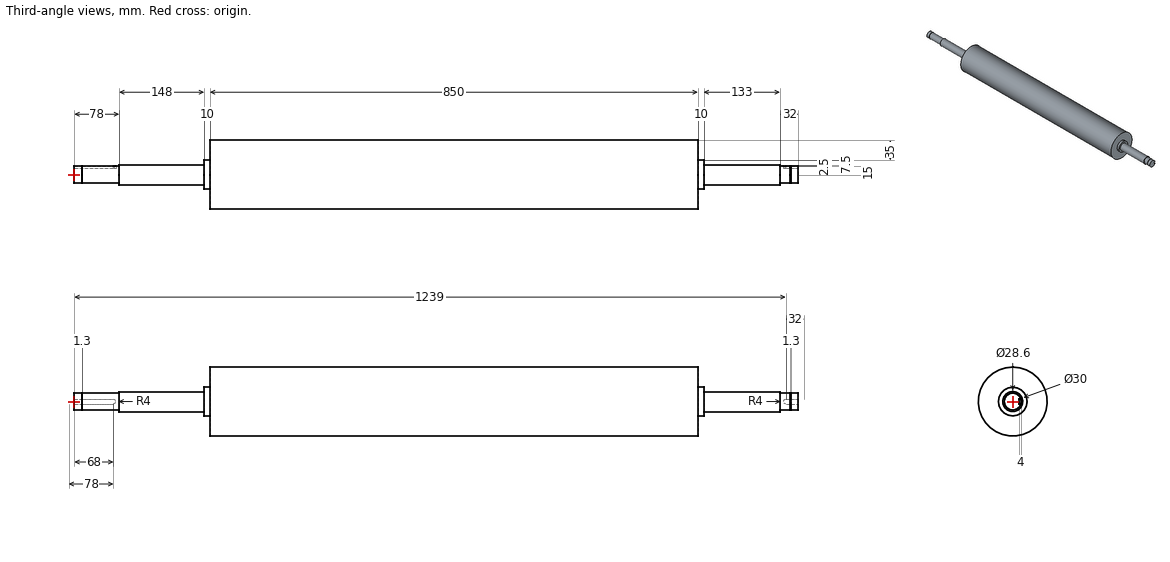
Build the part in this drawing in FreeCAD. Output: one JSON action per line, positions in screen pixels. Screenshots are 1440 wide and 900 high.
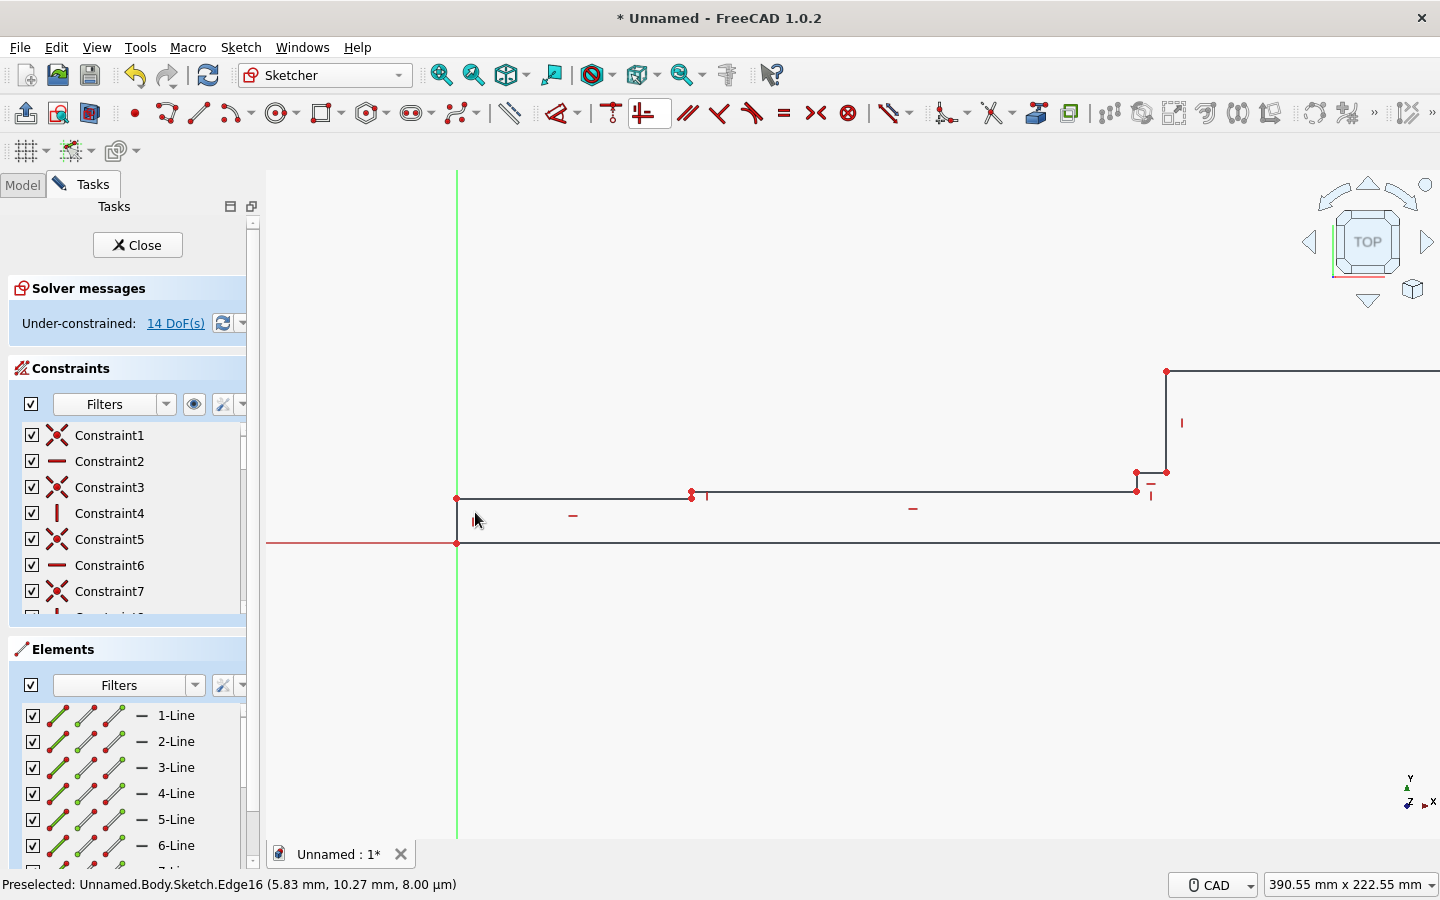
{"action": "scroll", "coordinate": [474, 515], "scroll_direction": "down", "scroll_amount": 9}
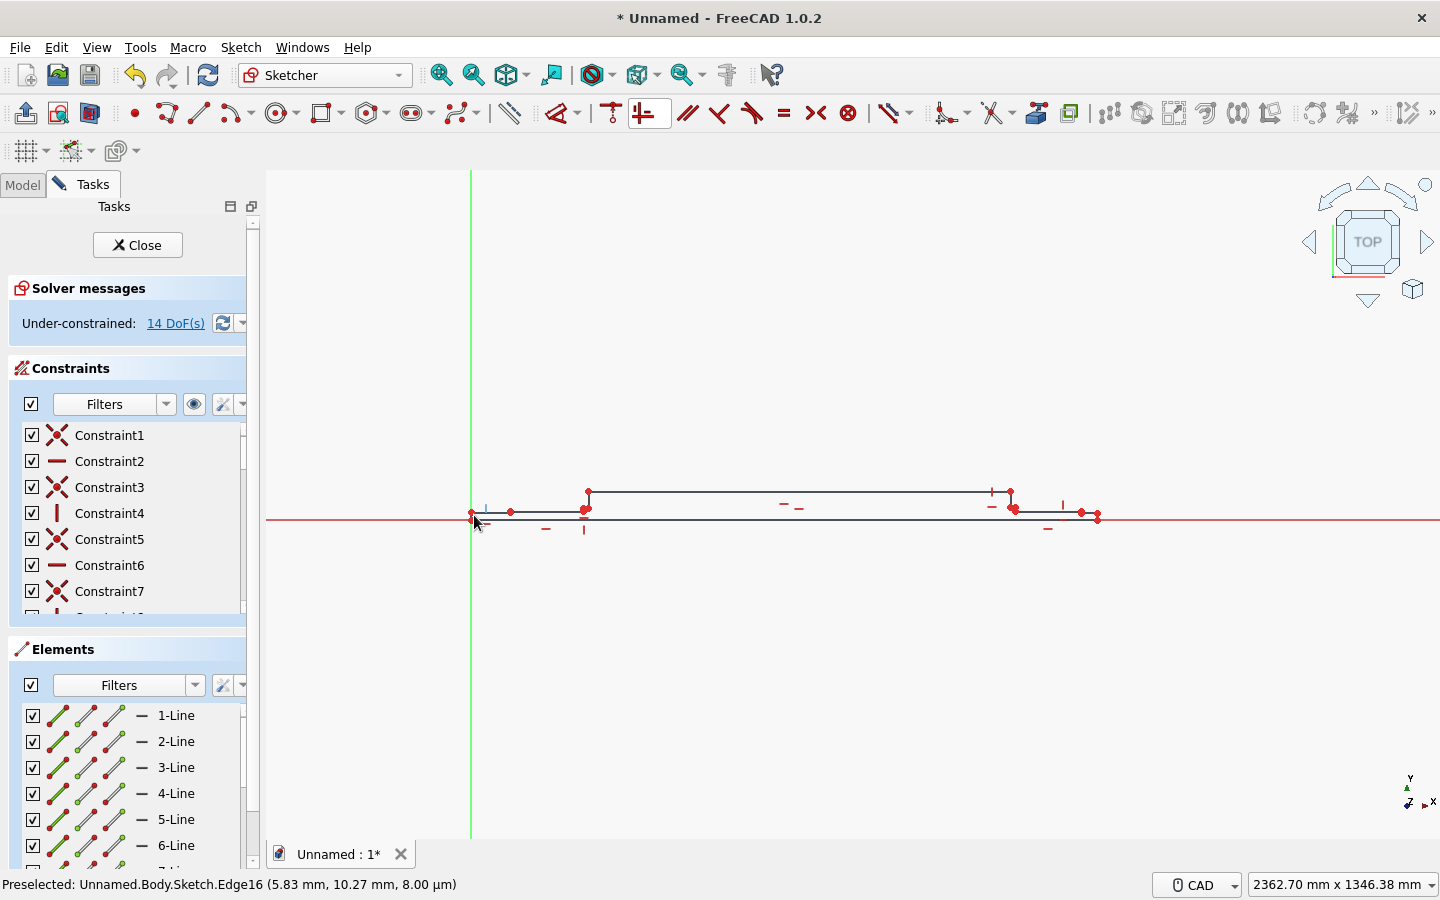
{"action": "scroll", "coordinate": [1098, 518], "scroll_direction": "up", "scroll_amount": 10}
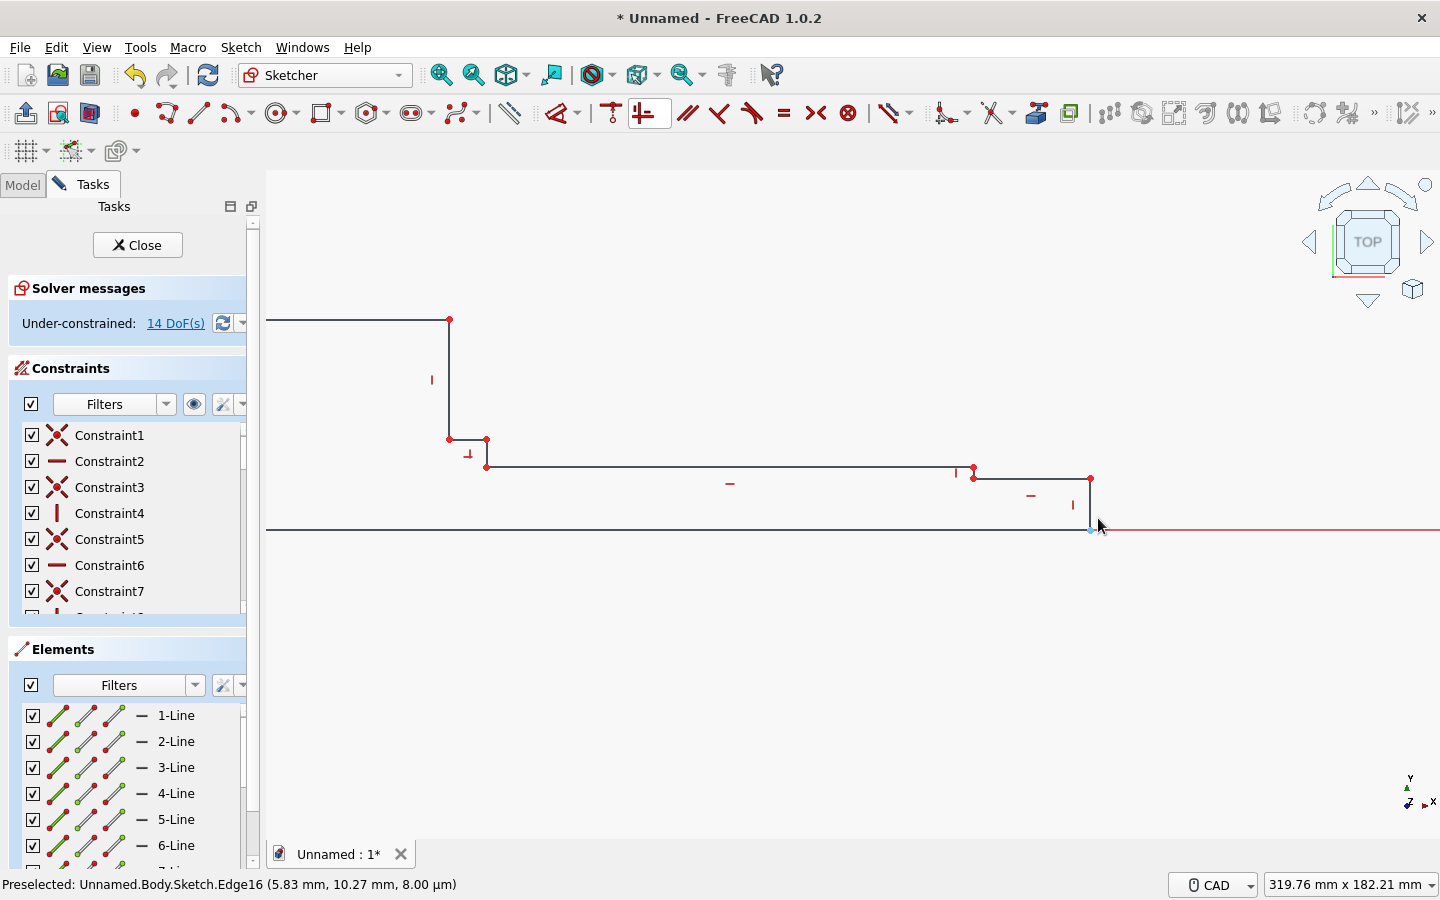
{"action": "left_click", "coordinate": [1090, 515]}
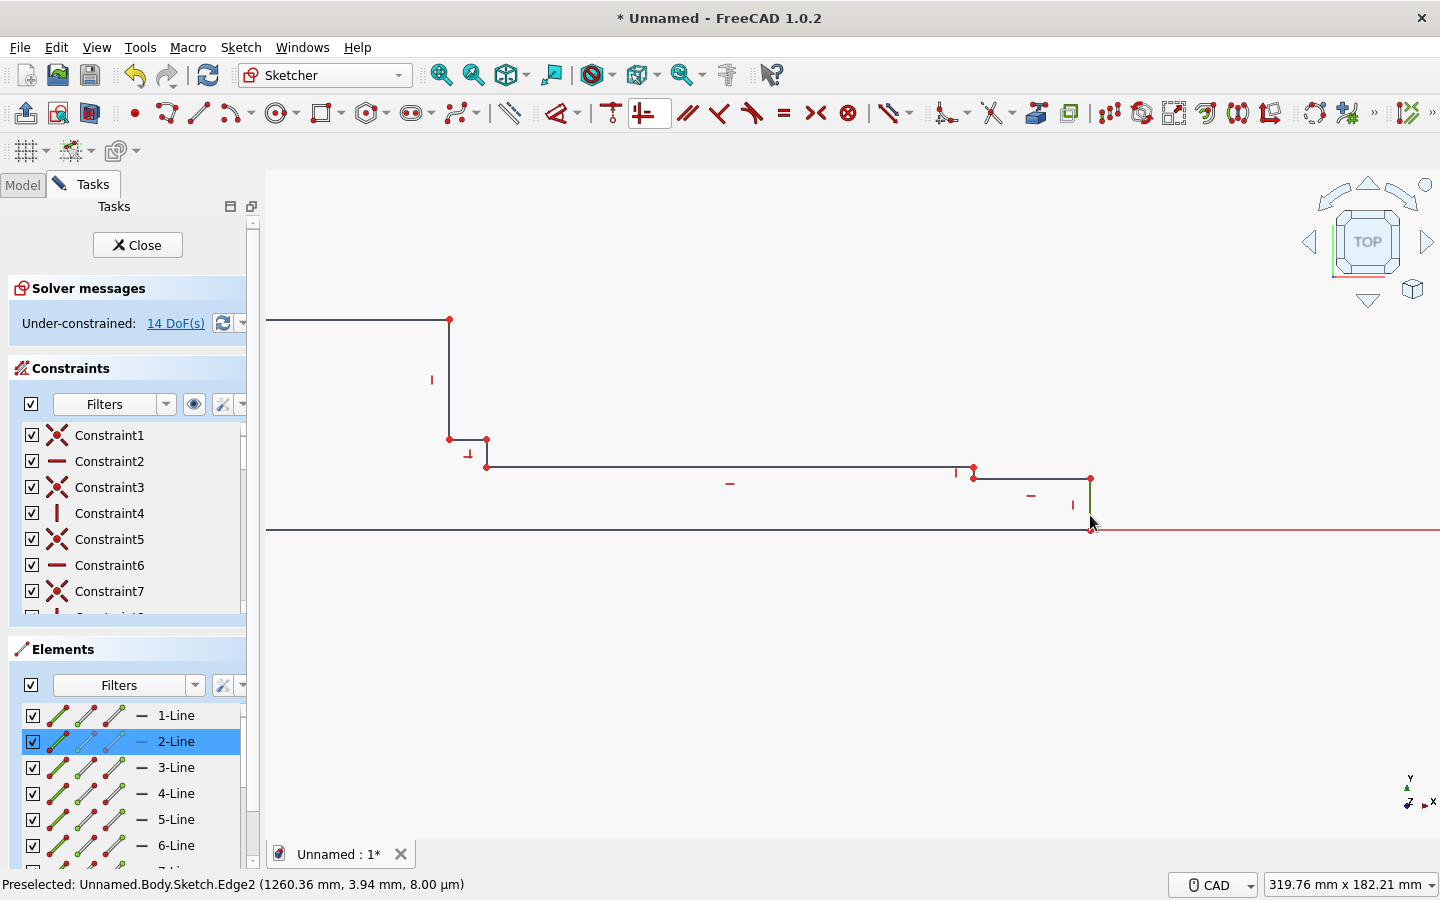
{"action": "left_click", "coordinate": [580, 114]}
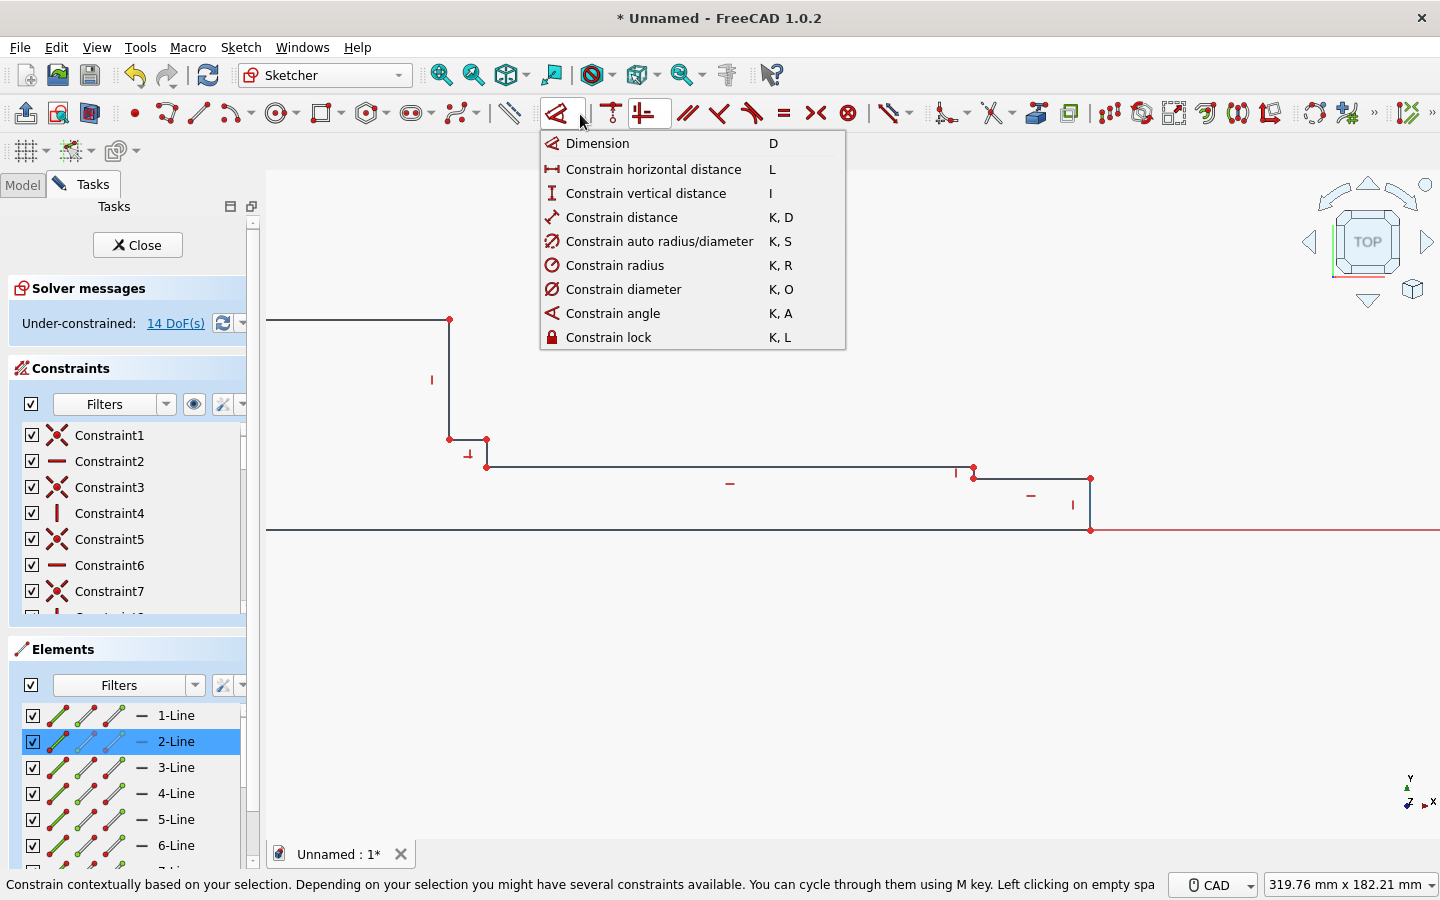
{"action": "left_click", "coordinate": [693, 193]}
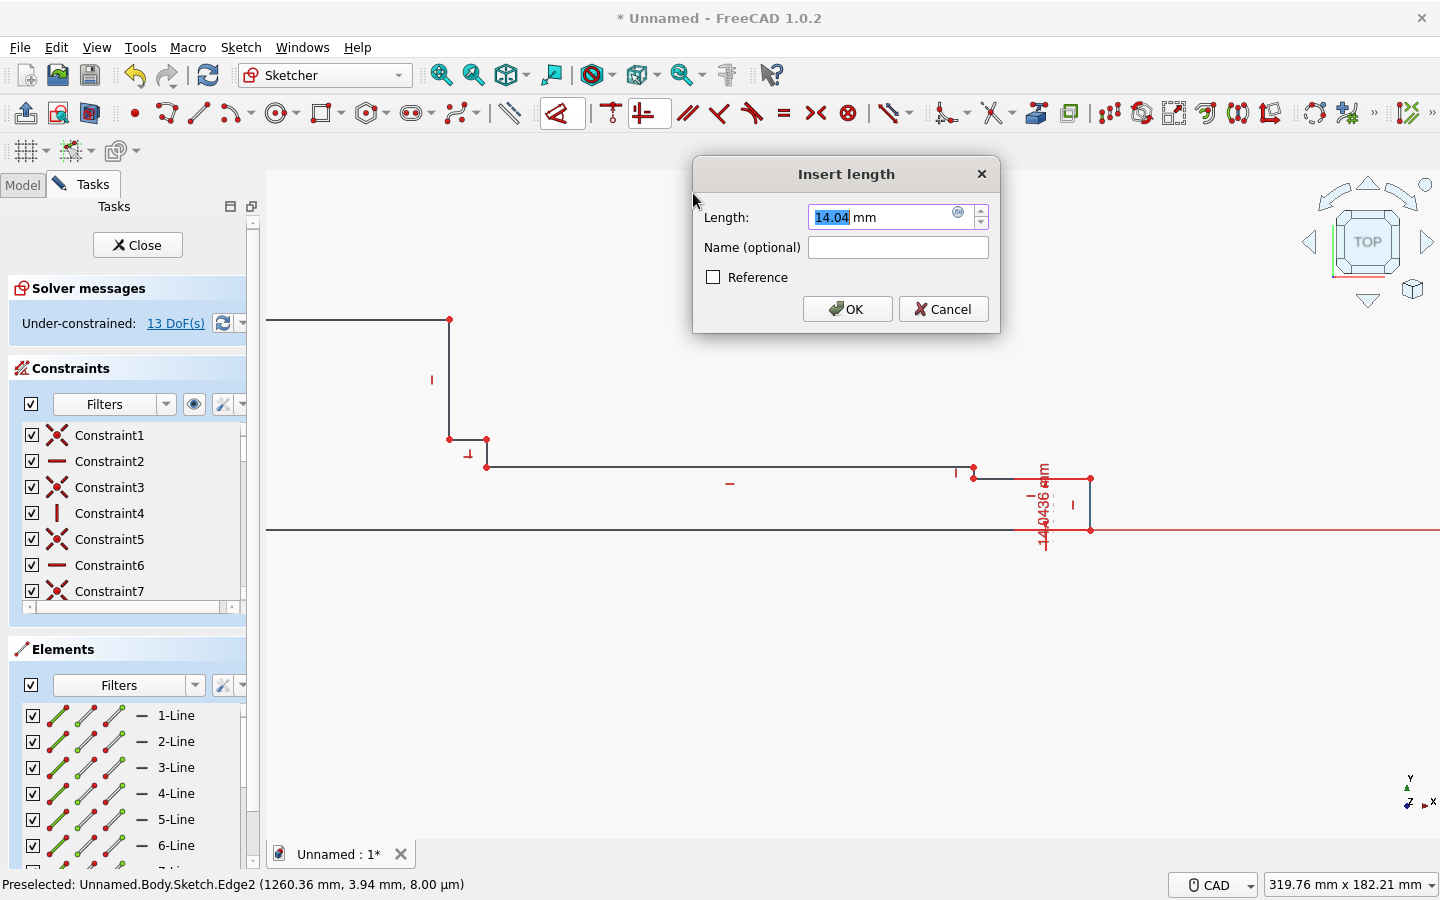
{"action": "type", "text": "15"}
{"action": "key", "text": "Return"}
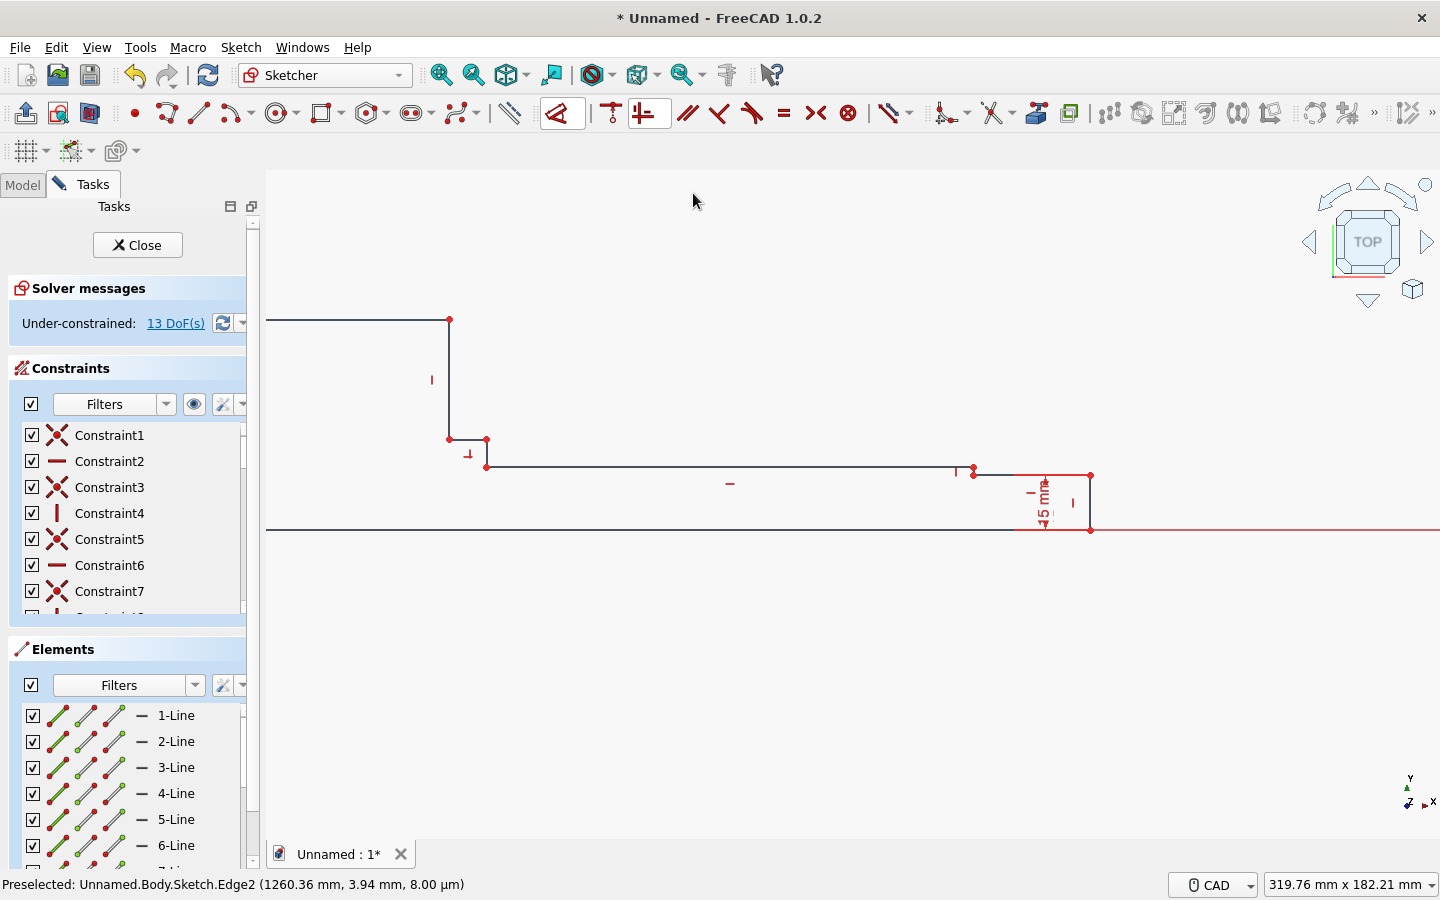
{"action": "left_click", "coordinate": [1055, 475]}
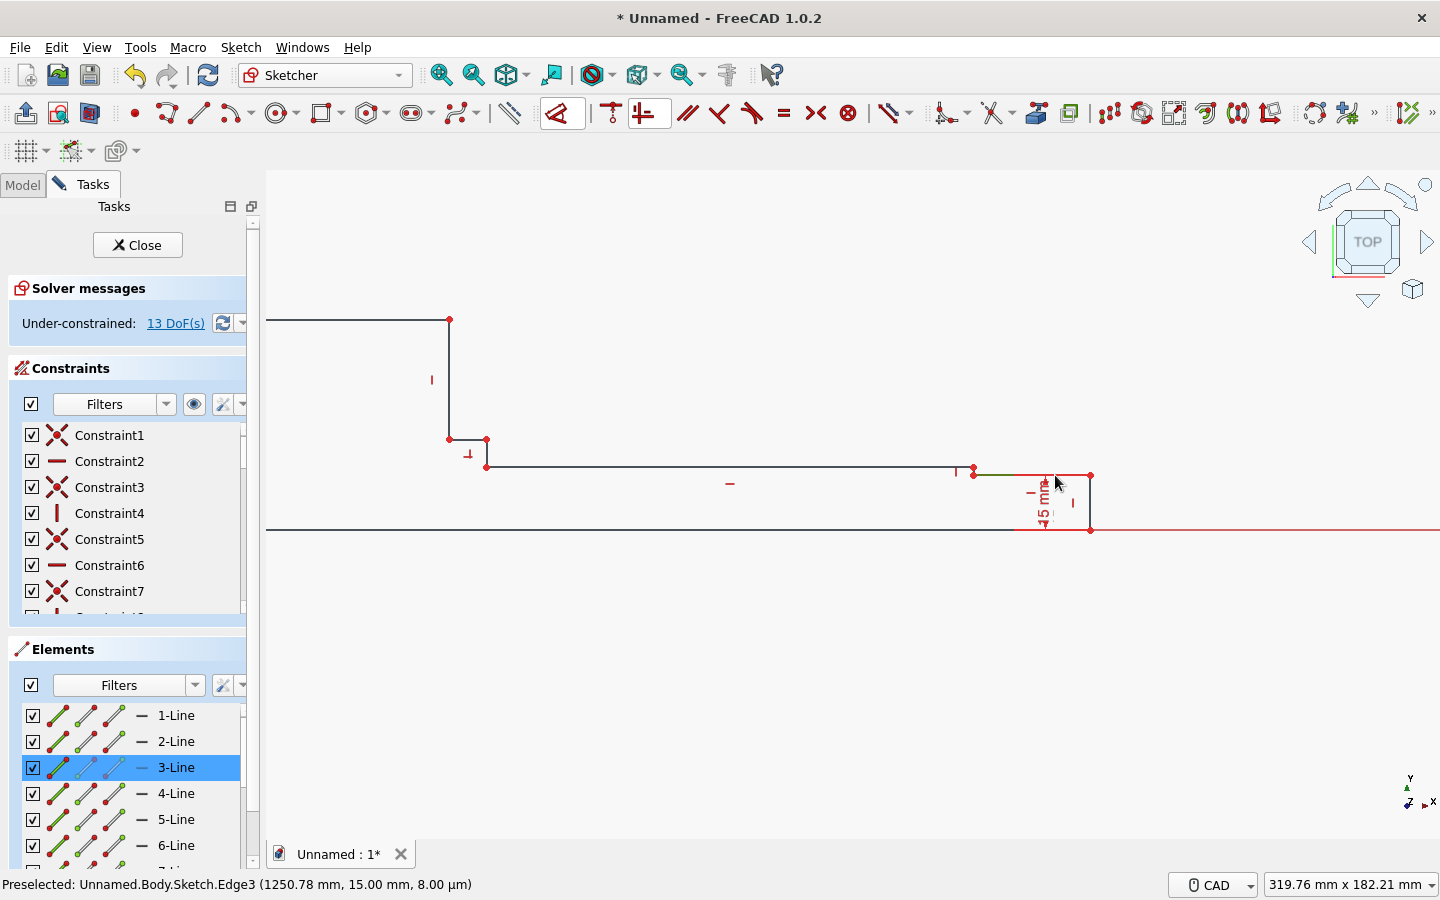
{"action": "key", "text": "l"}